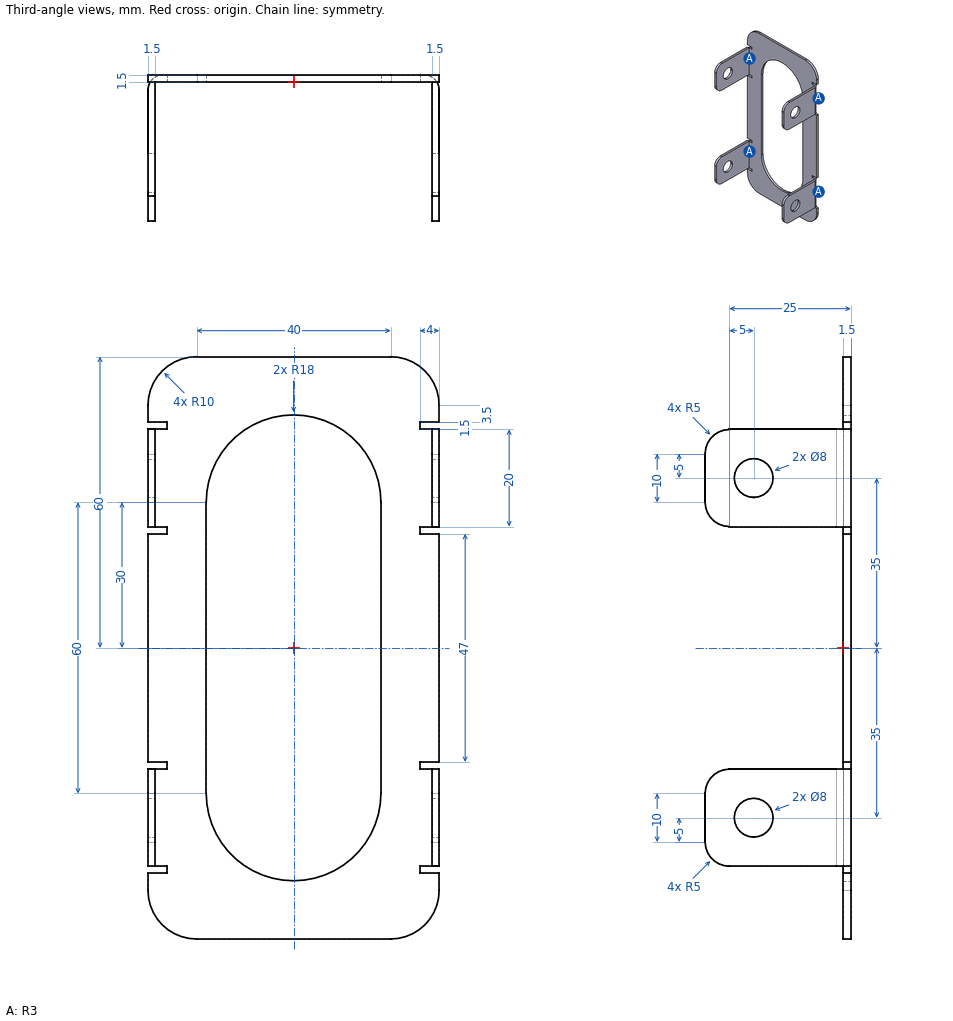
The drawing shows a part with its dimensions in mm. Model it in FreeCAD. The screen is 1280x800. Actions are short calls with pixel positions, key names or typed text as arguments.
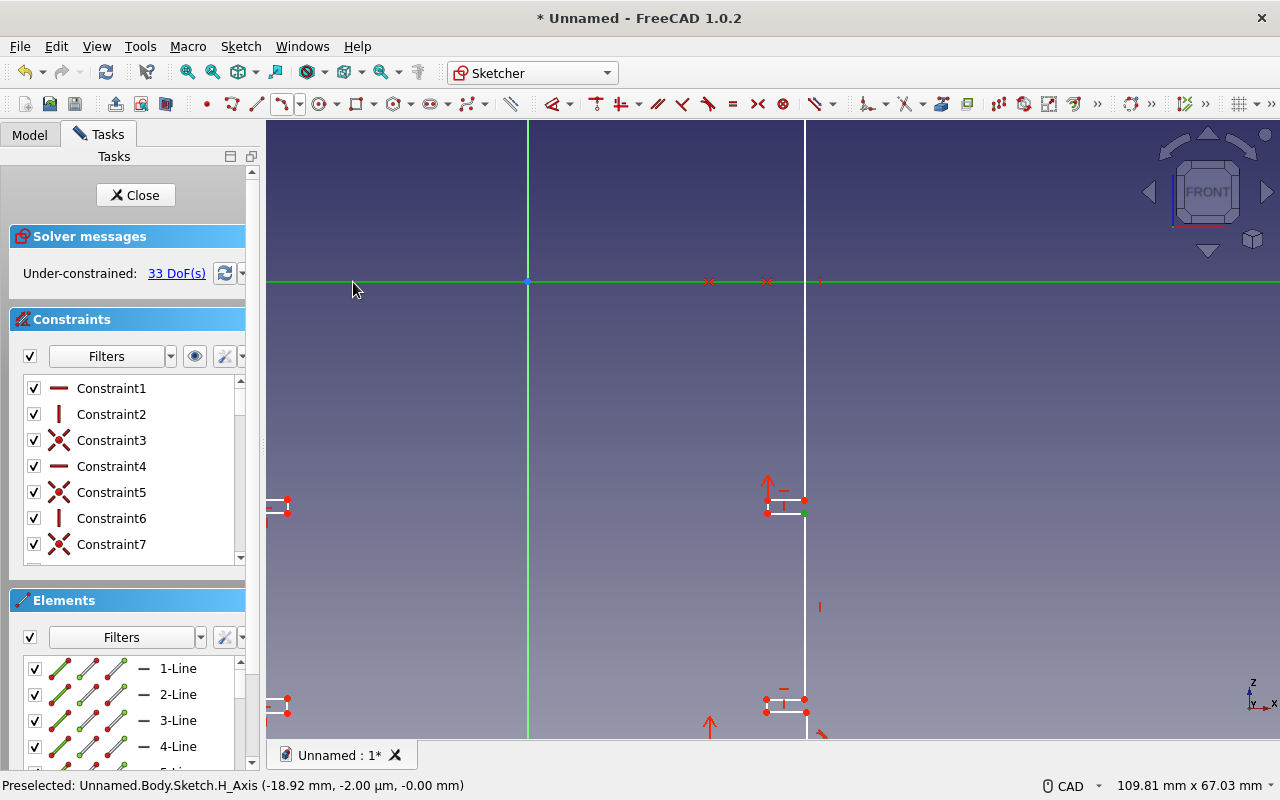
click(758, 104)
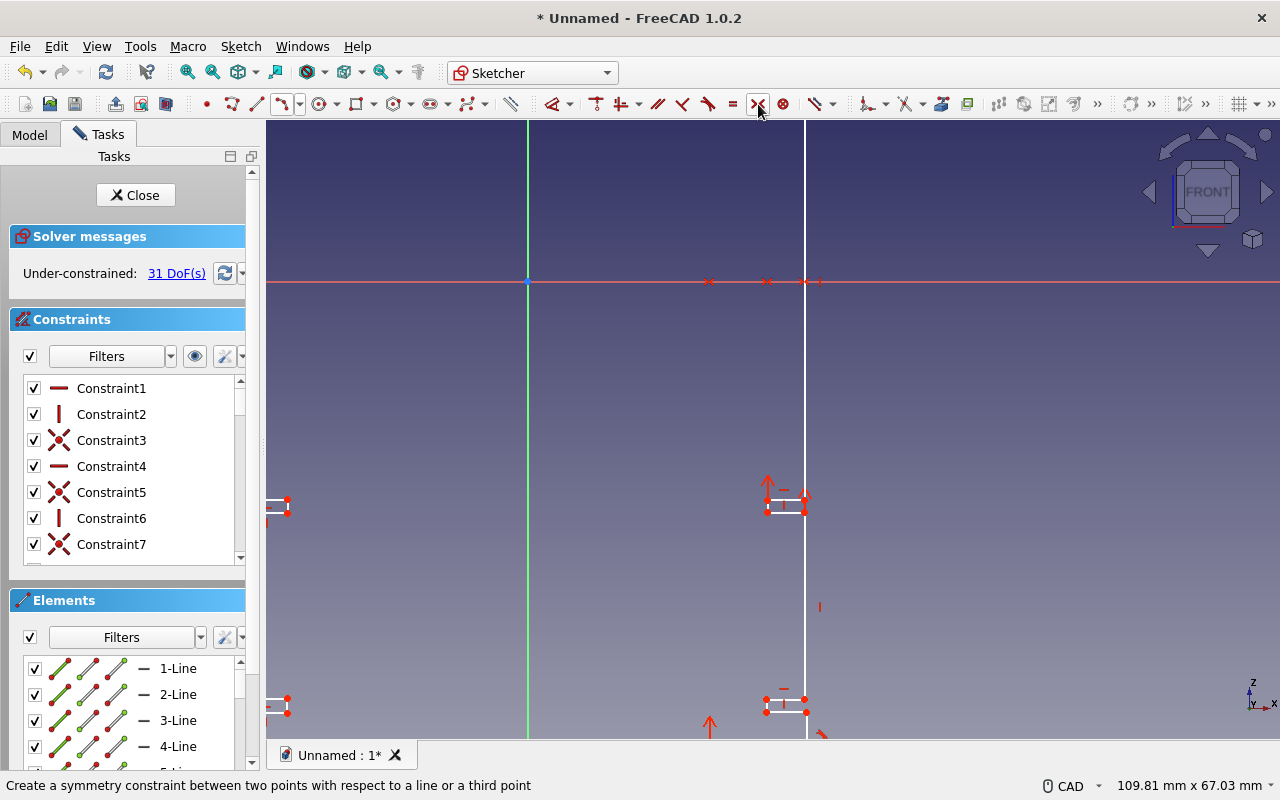
scroll(807, 515, down, 5)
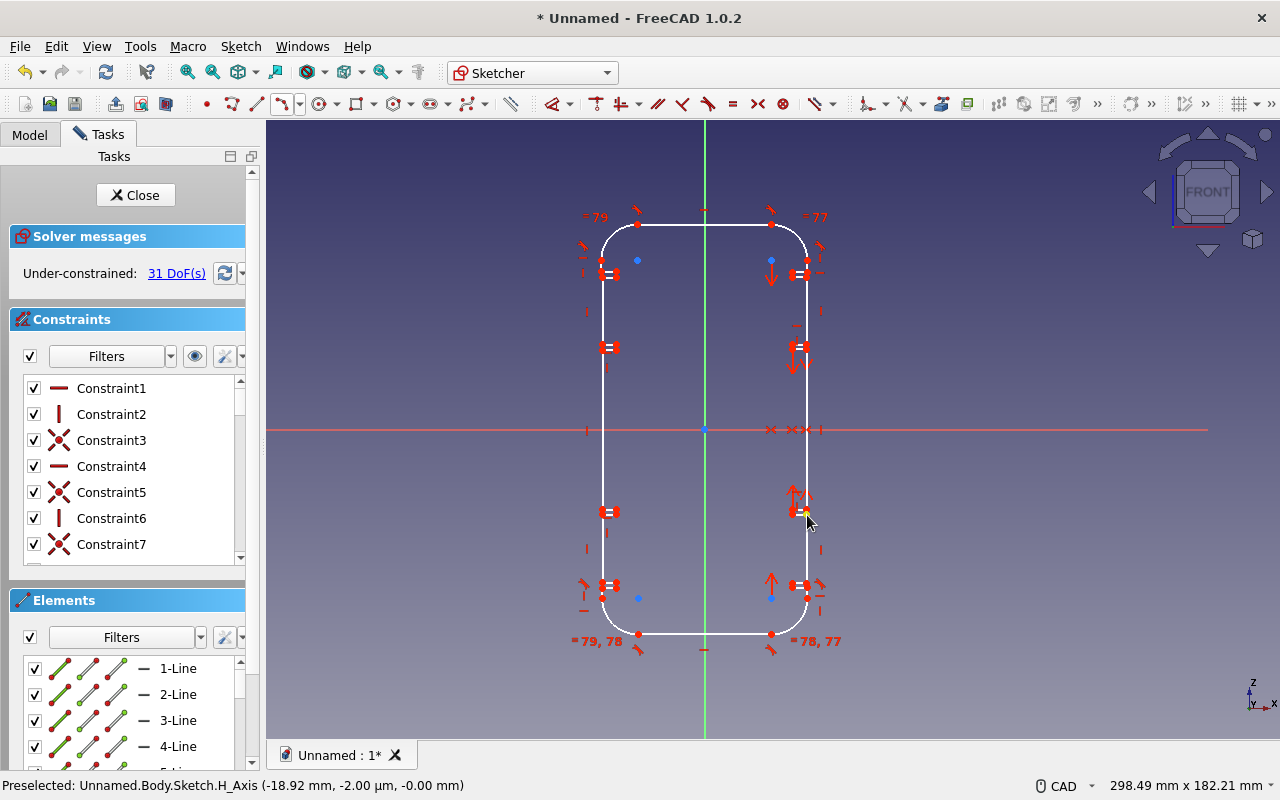
scroll(793, 277, up, 5)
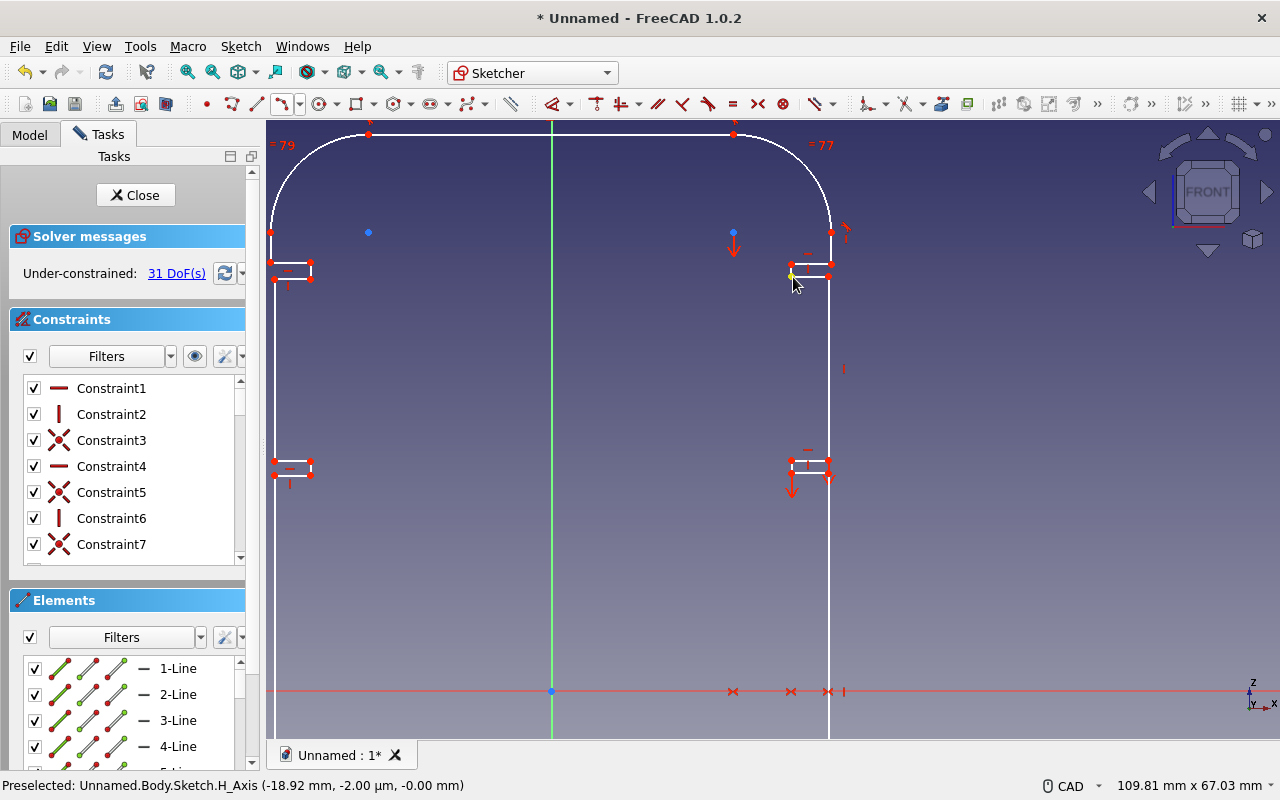
click(791, 277)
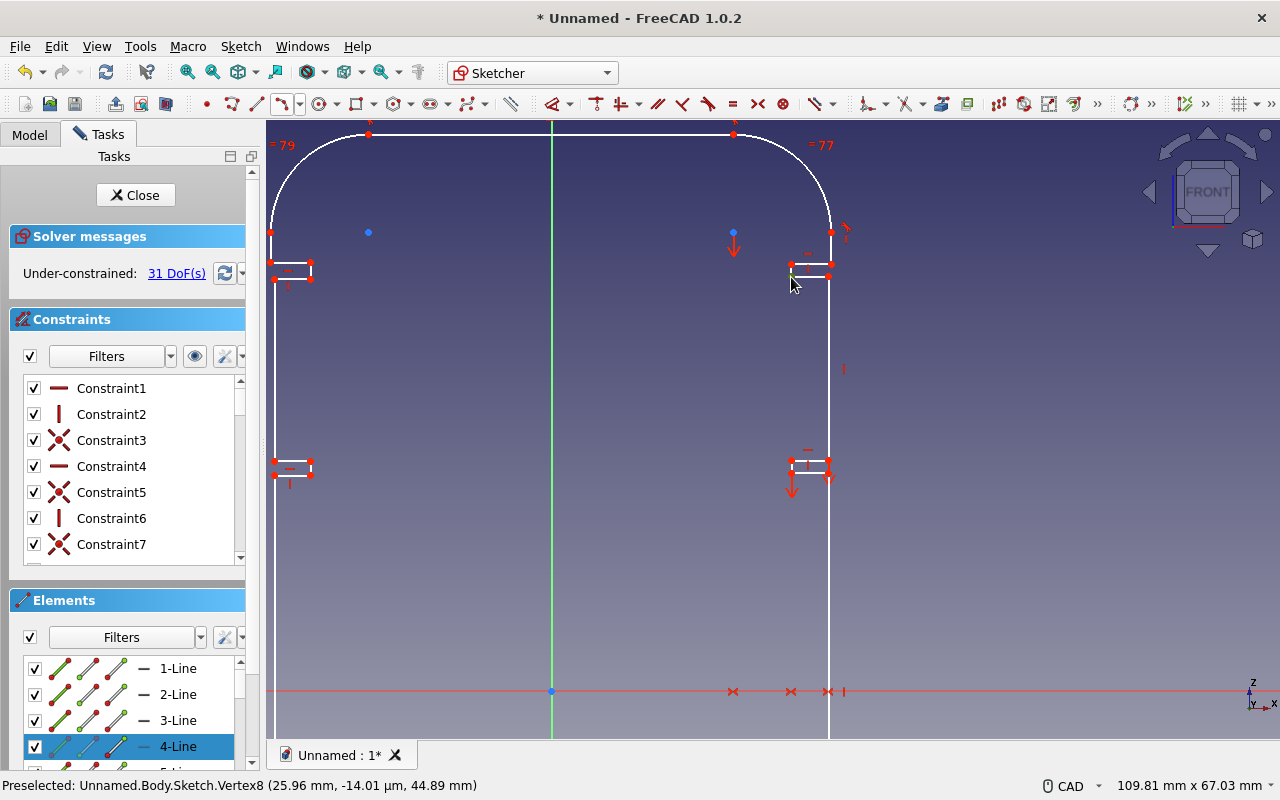
scroll(793, 277, down, 5)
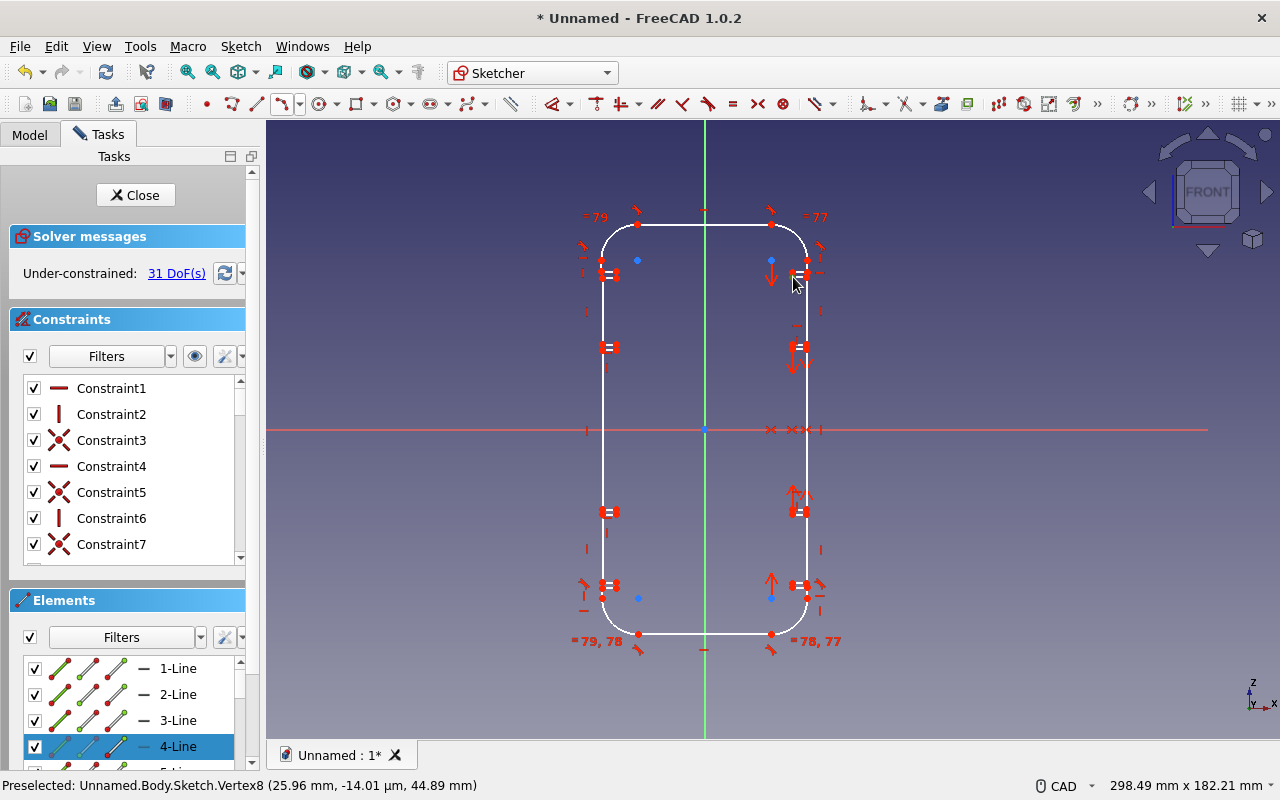
scroll(793, 583, up, 5)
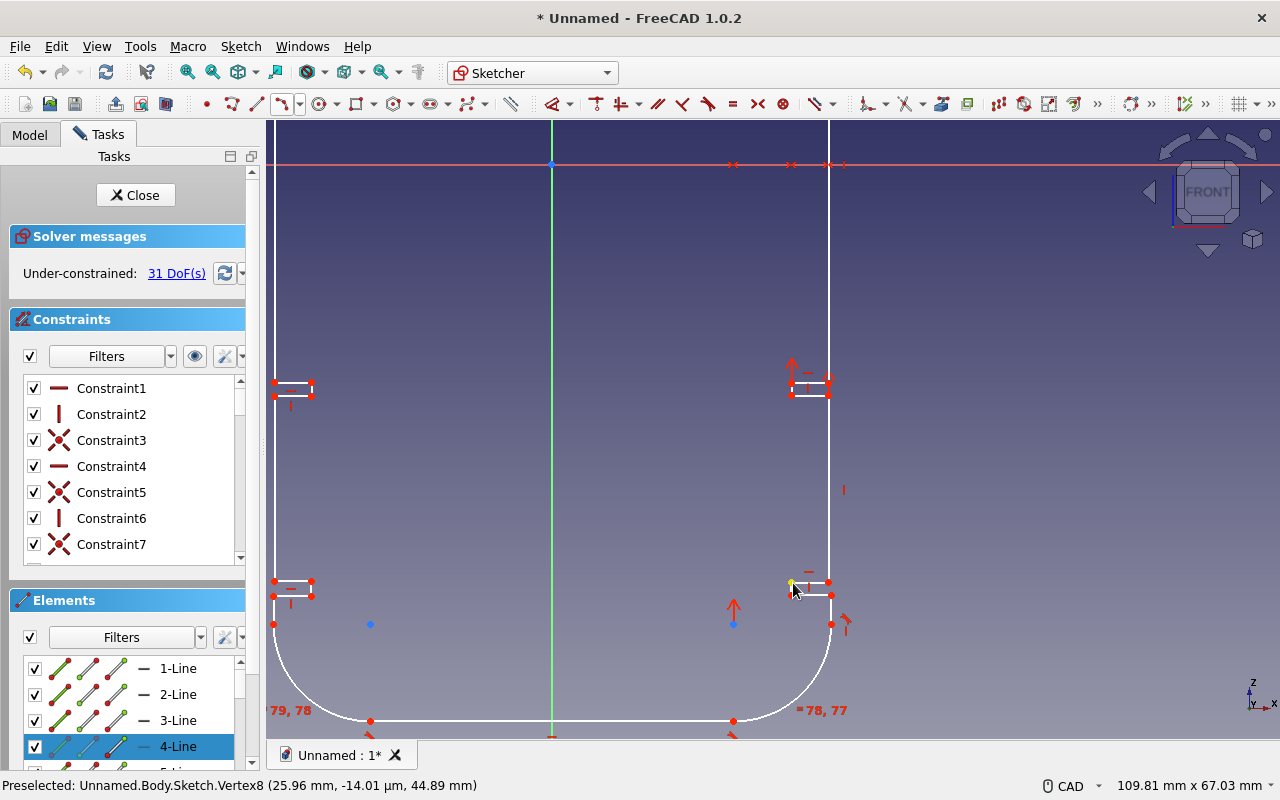
click(791, 583)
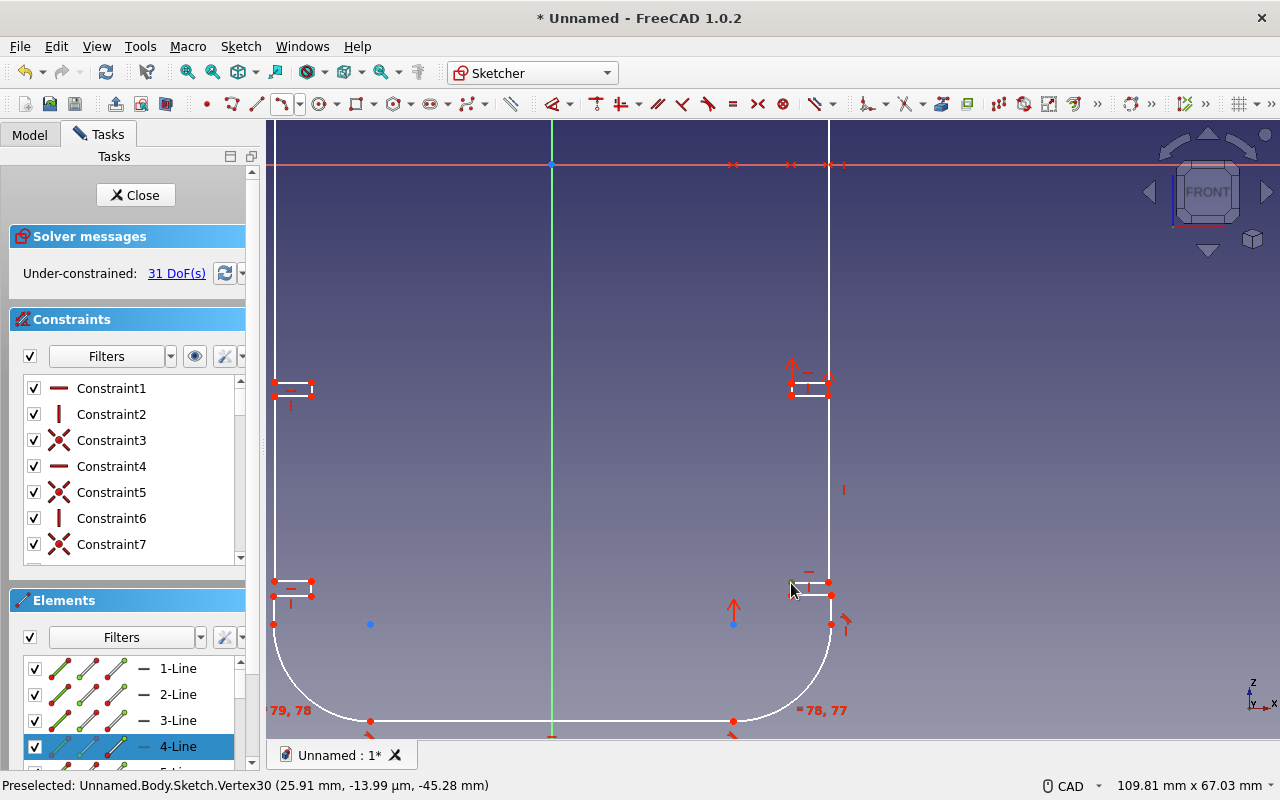
click(353, 165)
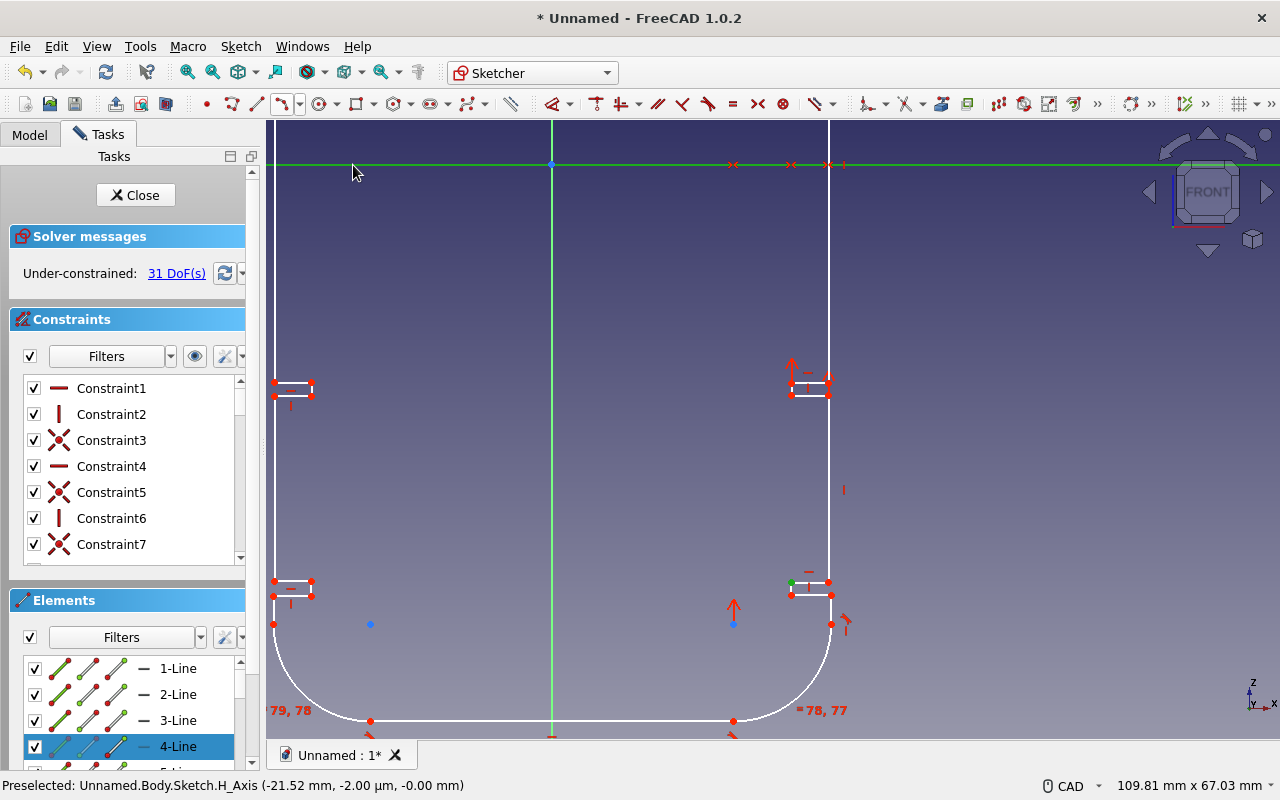
click(758, 104)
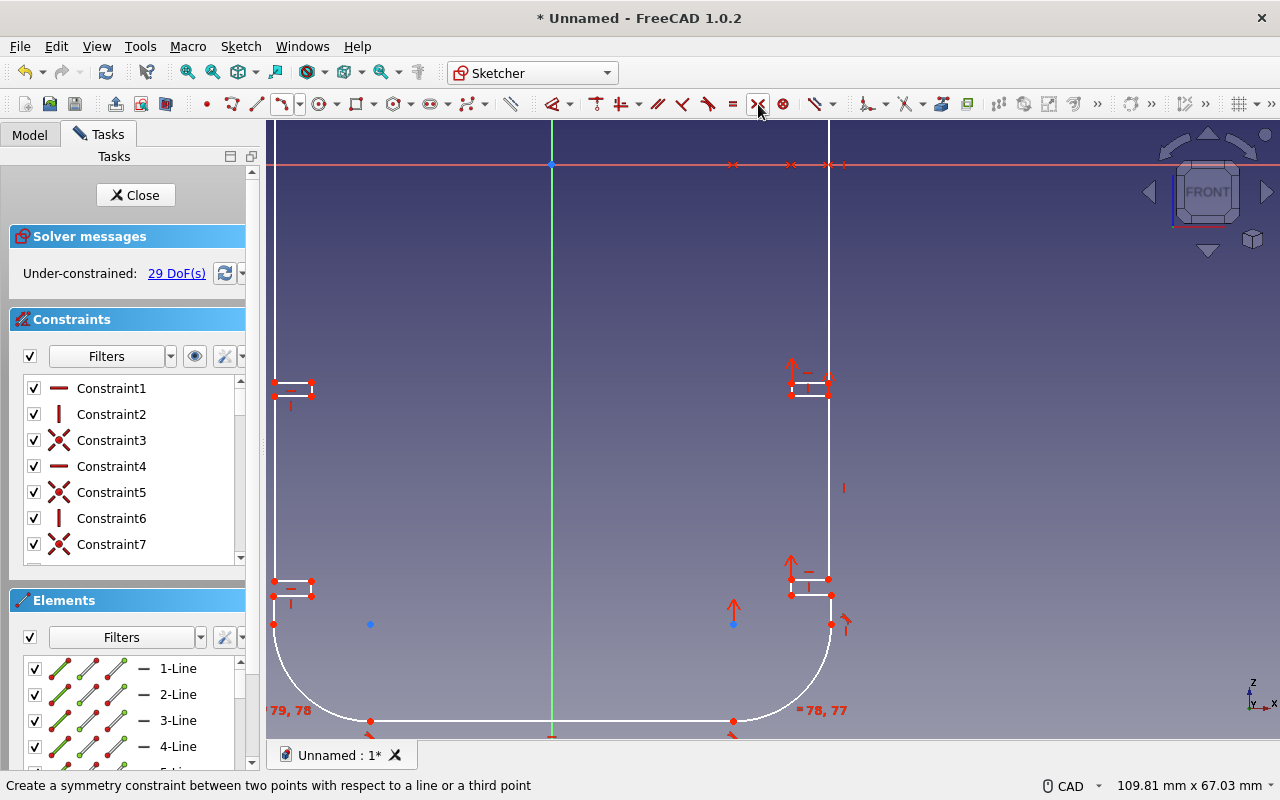
click(831, 595)